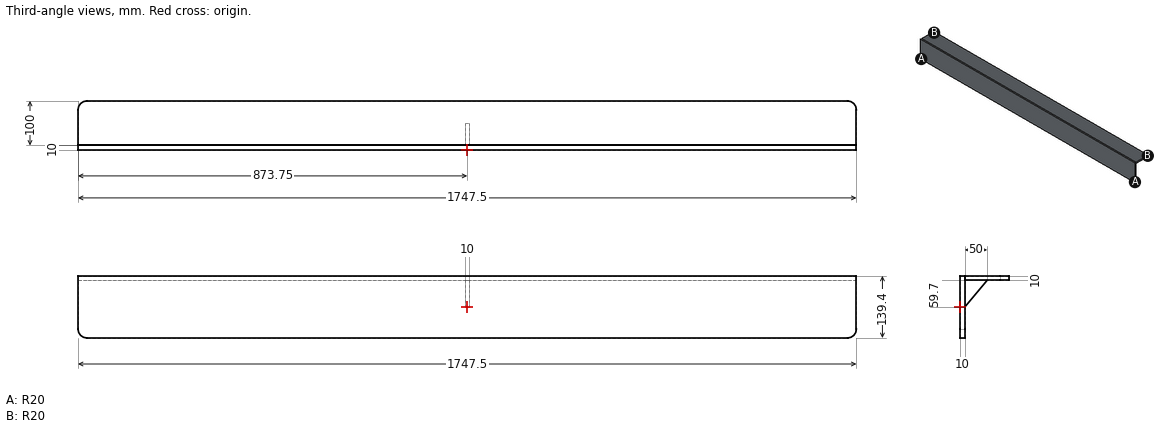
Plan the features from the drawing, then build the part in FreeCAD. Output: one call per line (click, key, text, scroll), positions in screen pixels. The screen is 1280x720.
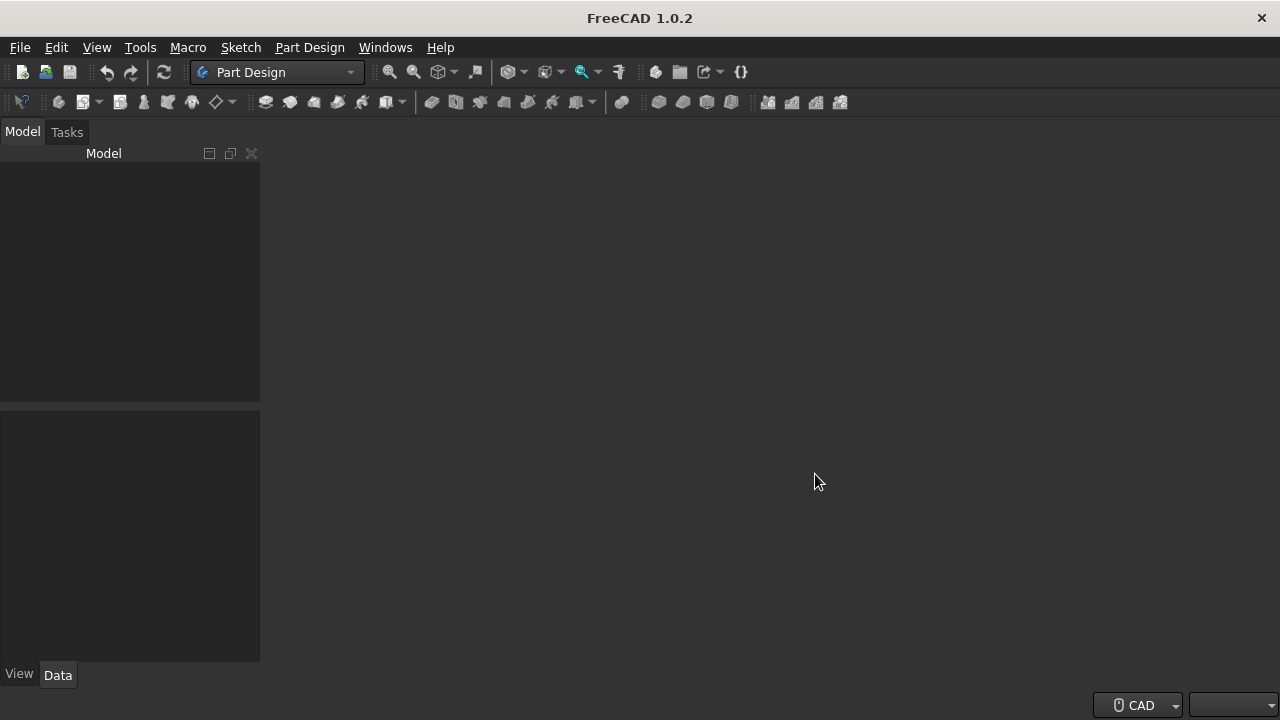
click(22, 72)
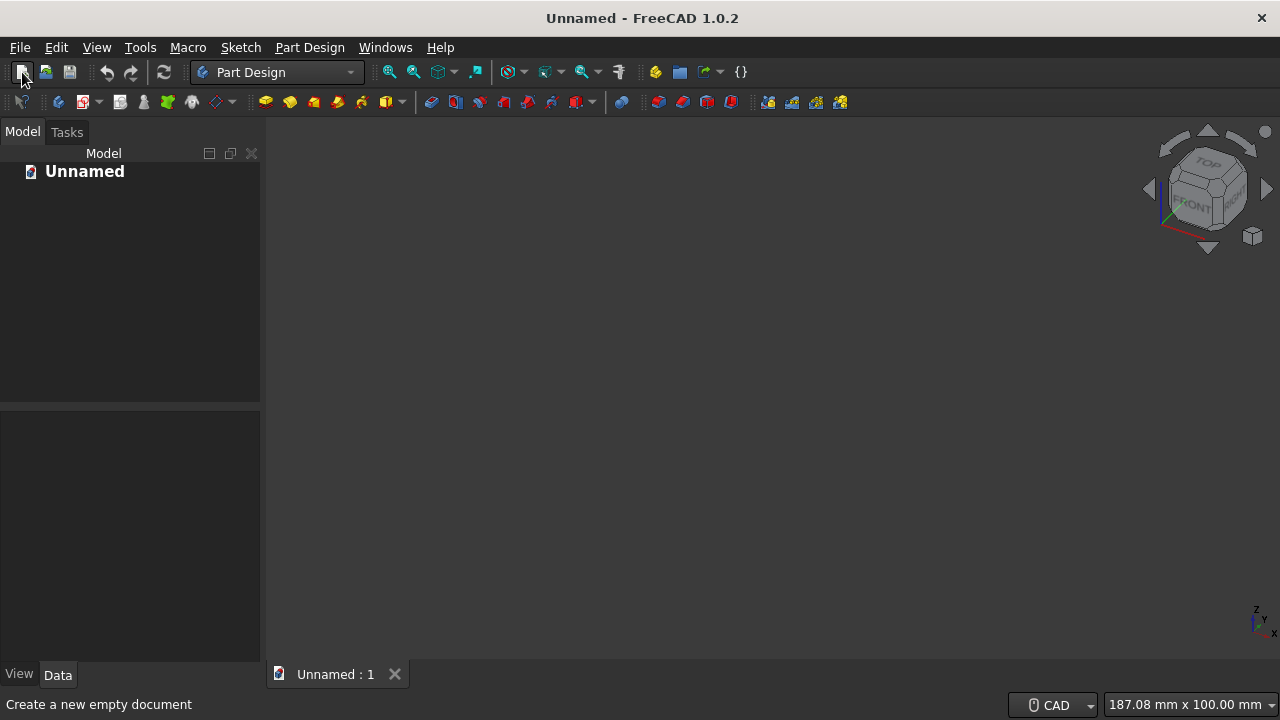
click(84, 102)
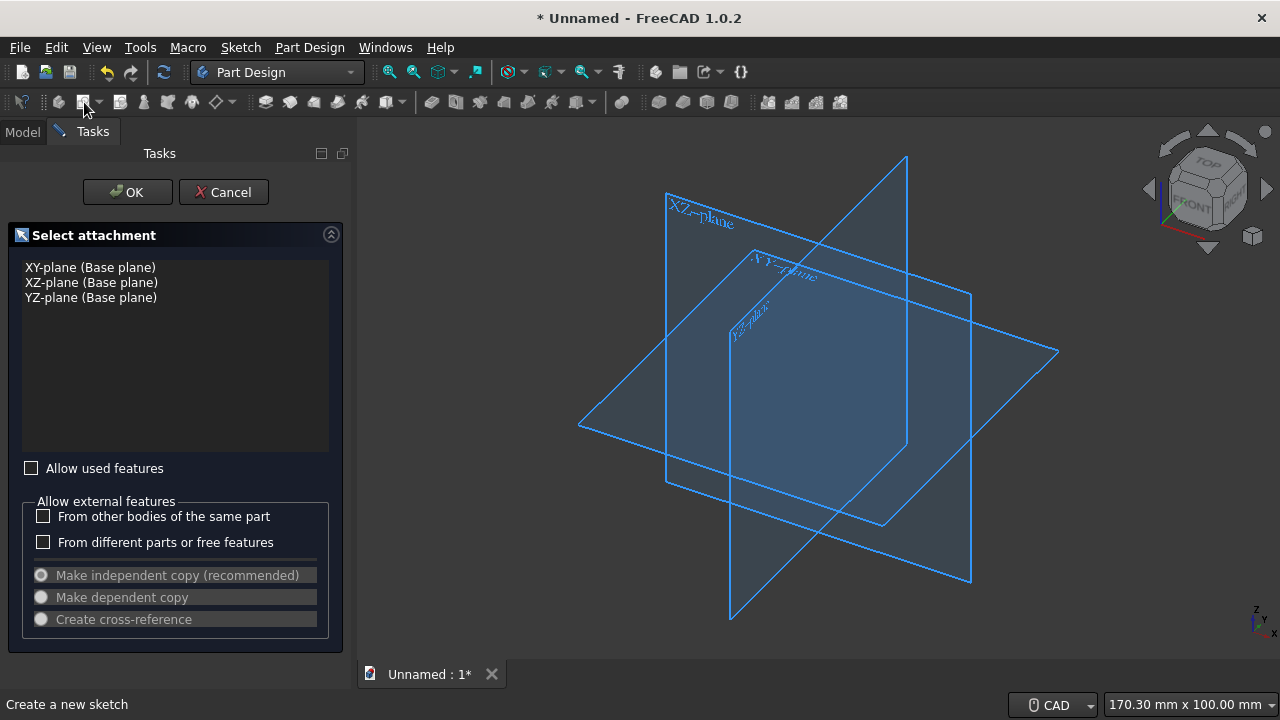
click(82, 282)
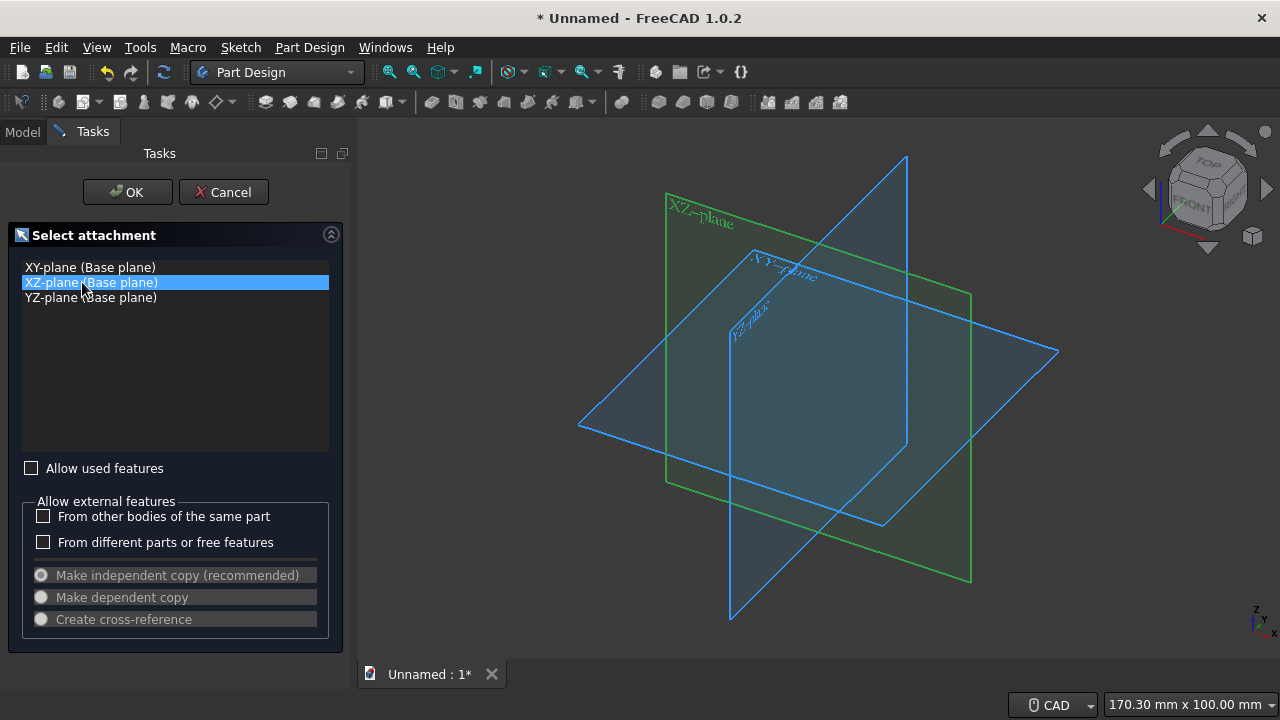
click(128, 192)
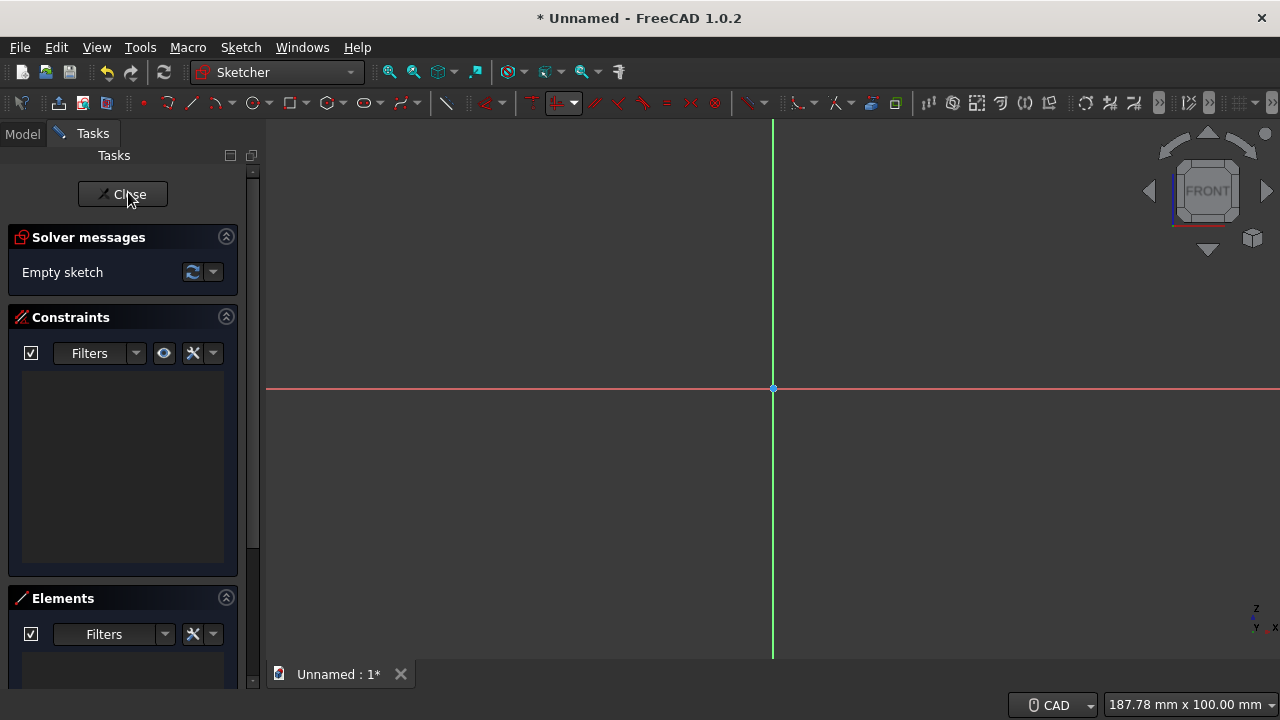
scroll(700, 389, down, 14)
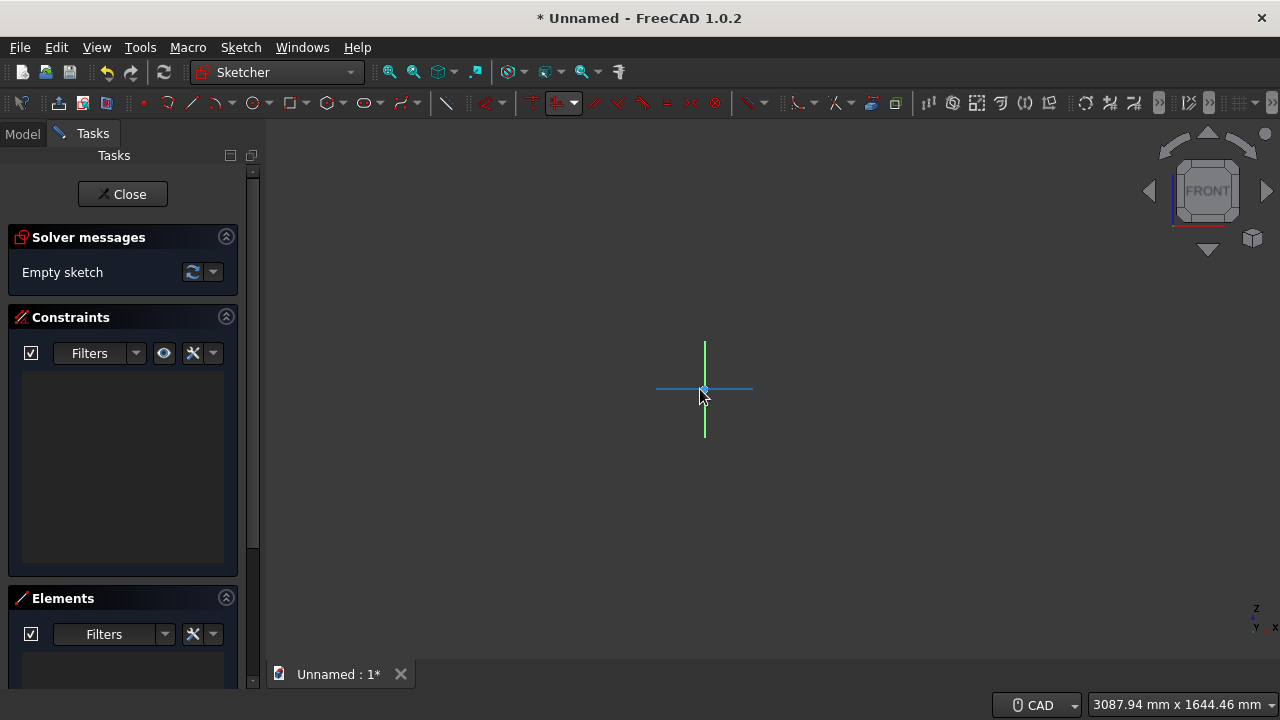
key(g)
key(v)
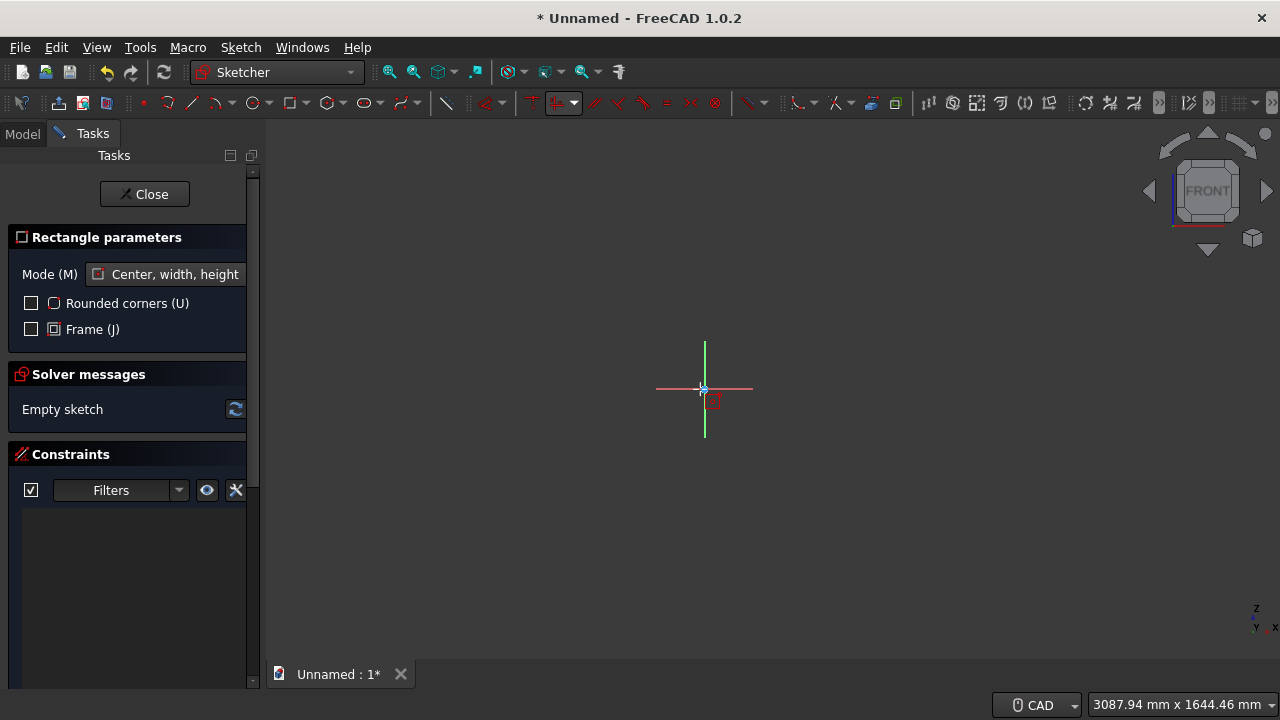
click(705, 389)
click(992, 367)
key(Escape)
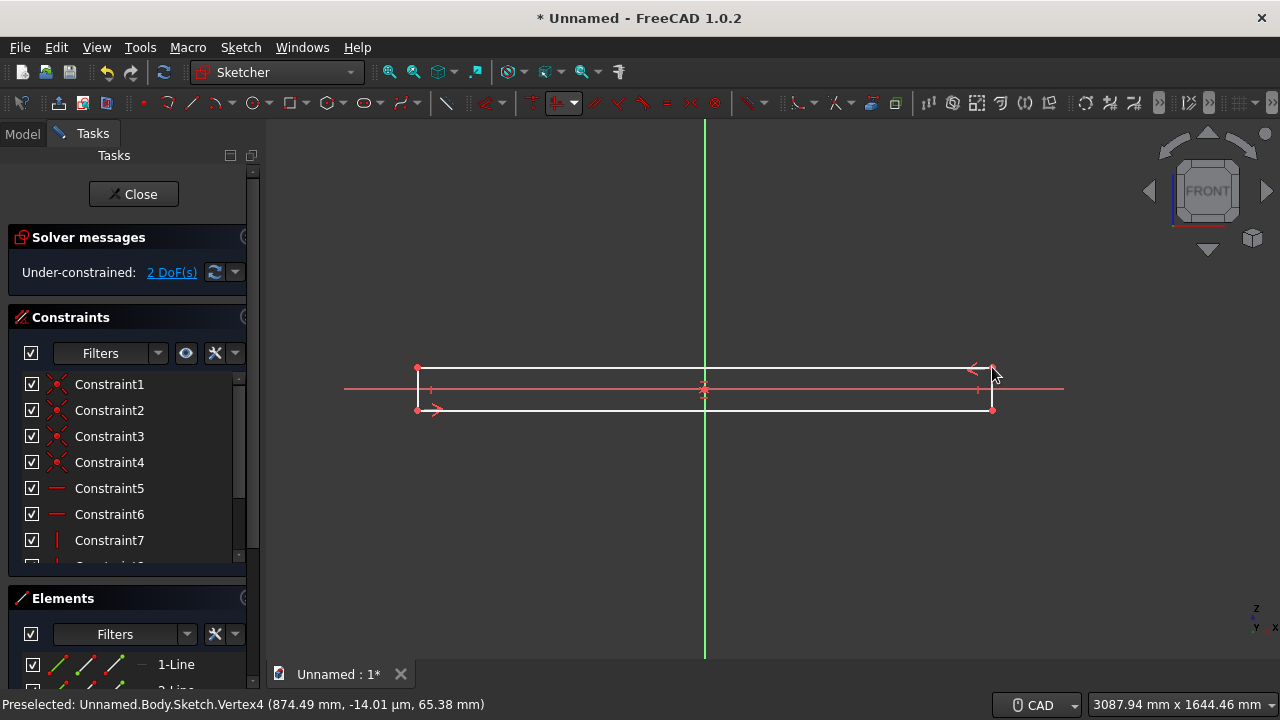
click(992, 389)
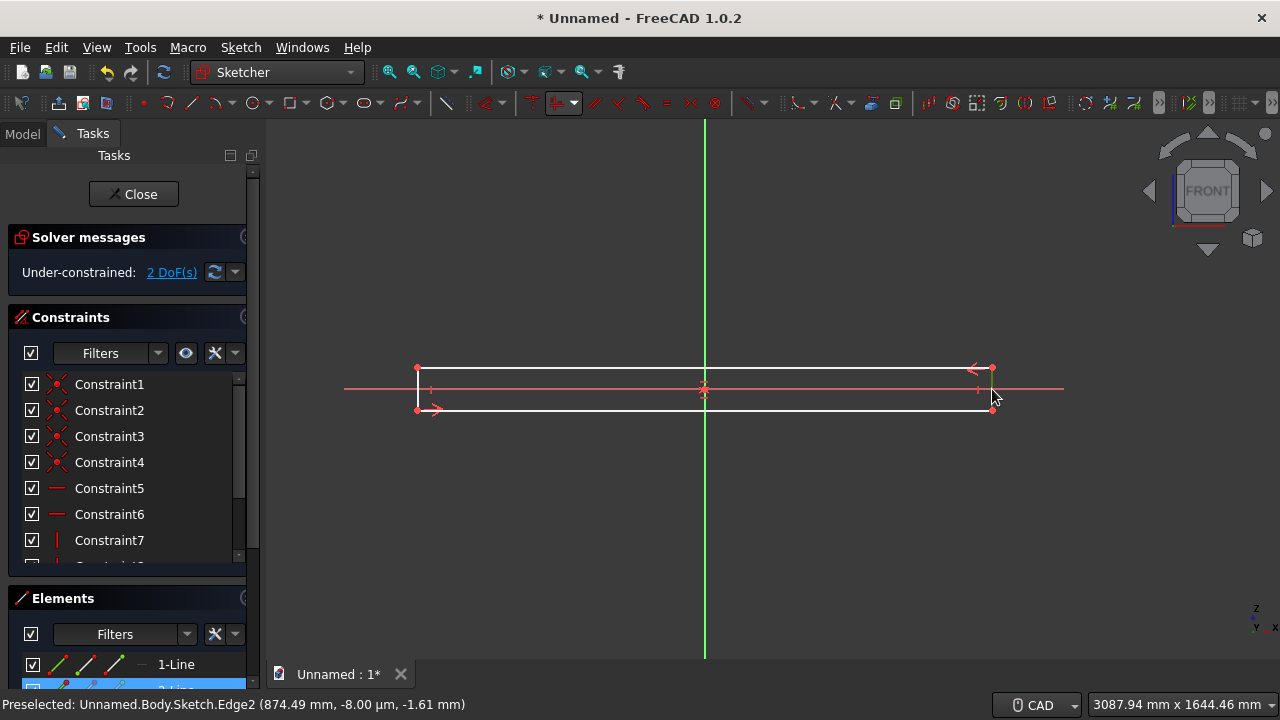
click(504, 104)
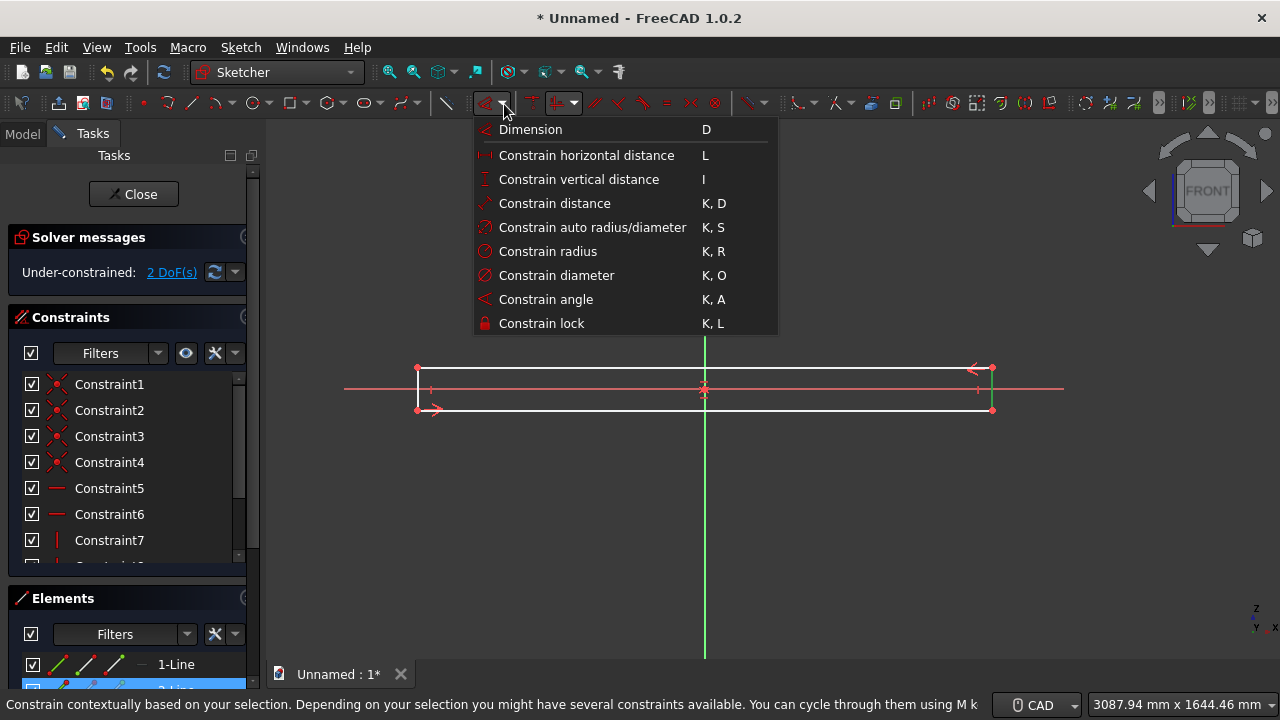
click(626, 179)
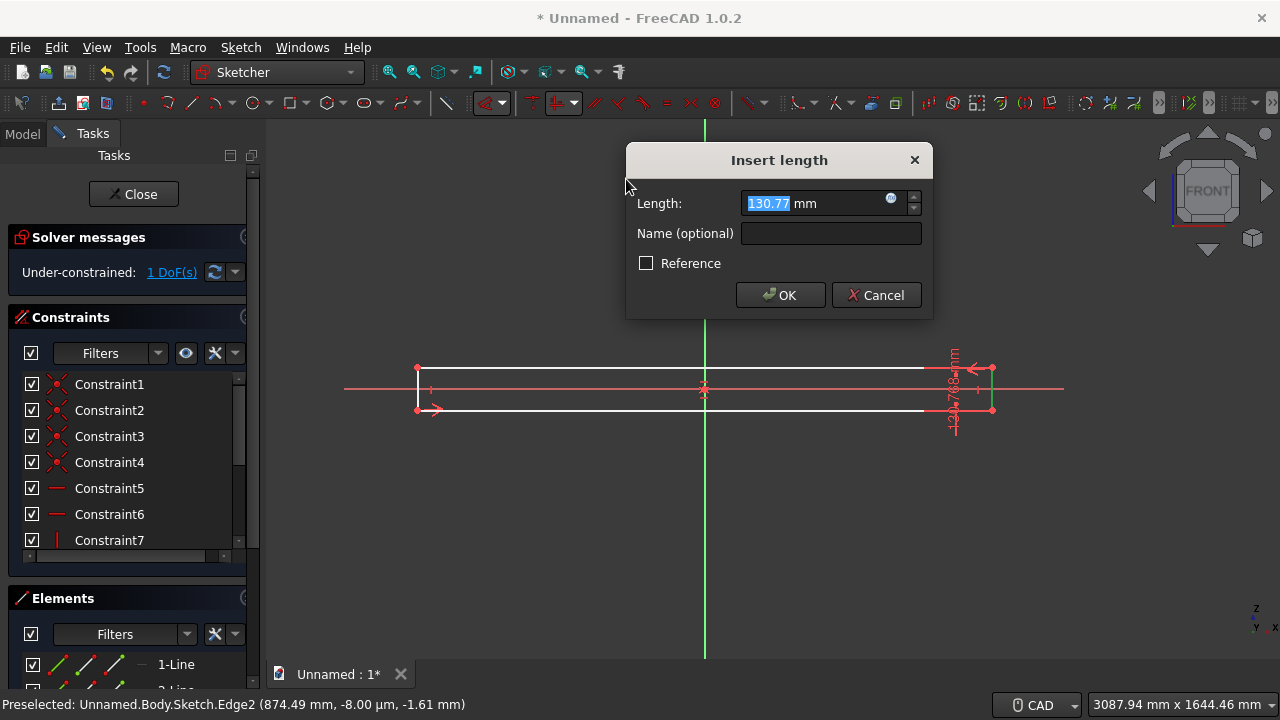
text(139.4)
key(Return)